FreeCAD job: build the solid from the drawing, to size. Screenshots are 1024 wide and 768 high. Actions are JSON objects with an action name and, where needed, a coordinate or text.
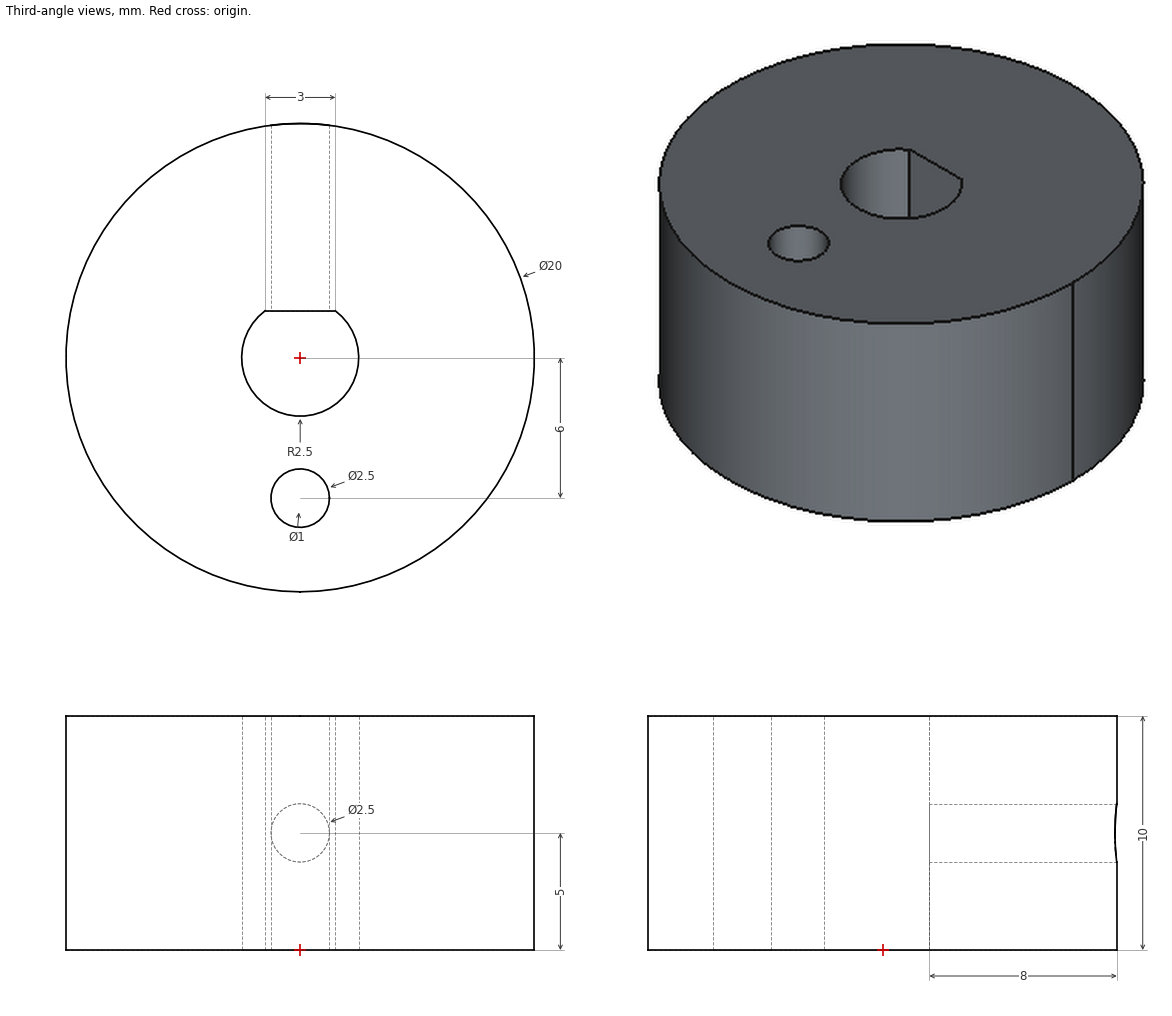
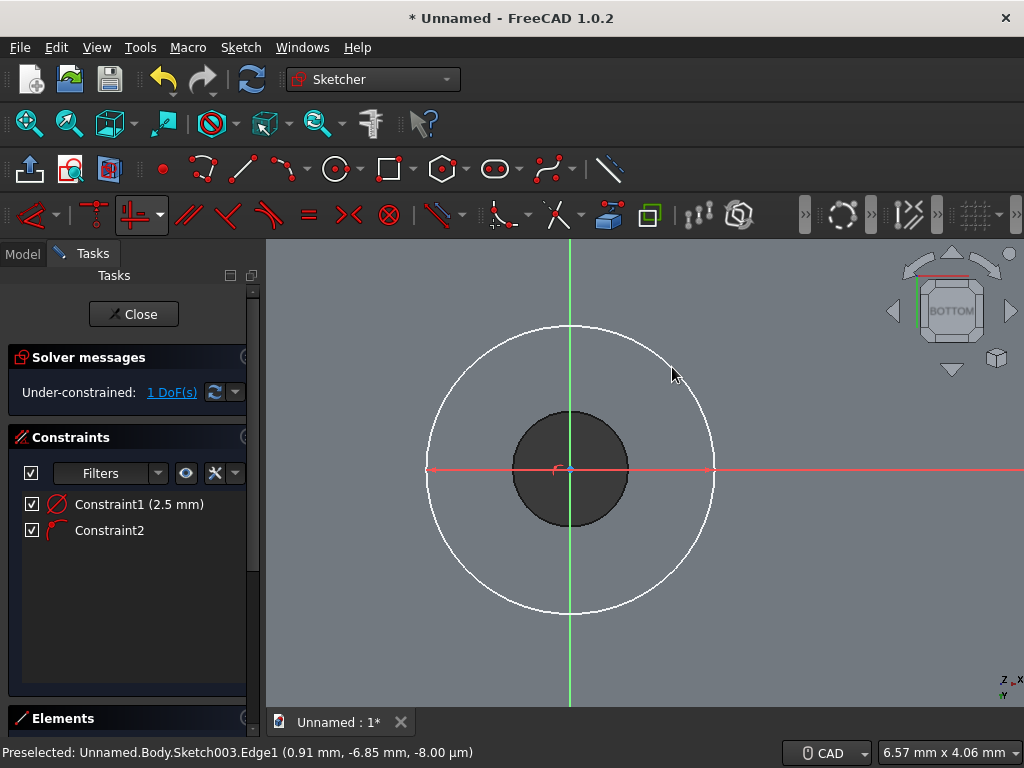
{"action": "left_click", "coordinate": [32, 216]}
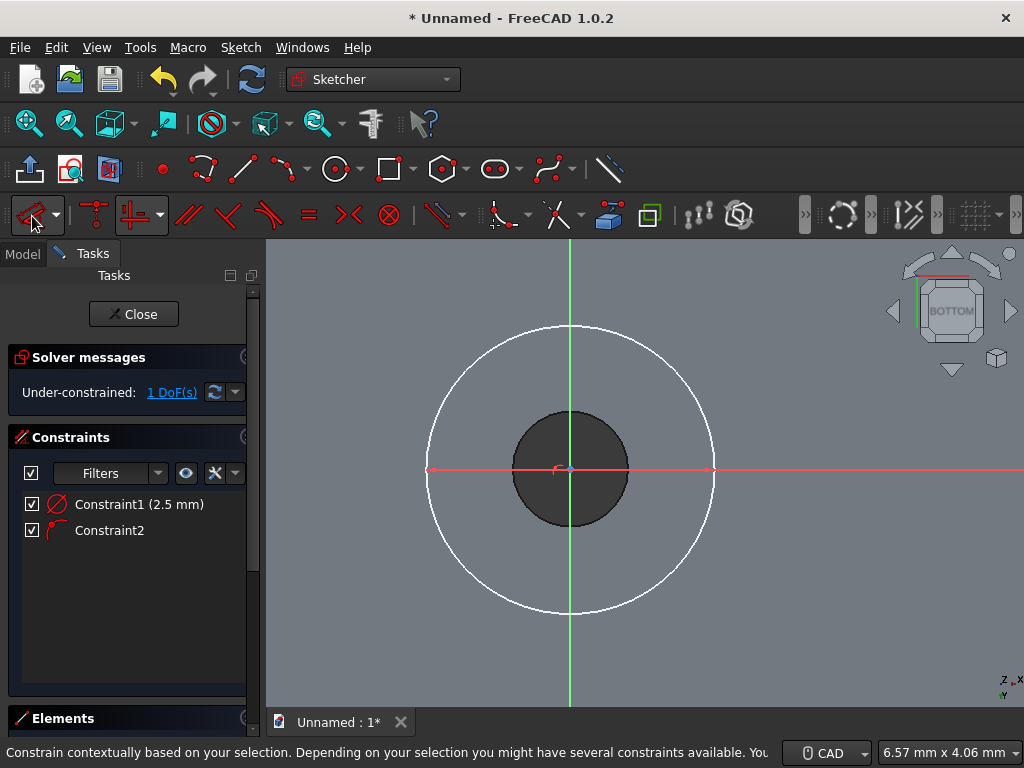
{"action": "left_click", "coordinate": [570, 470]}
{"action": "left_click", "coordinate": [604, 574]}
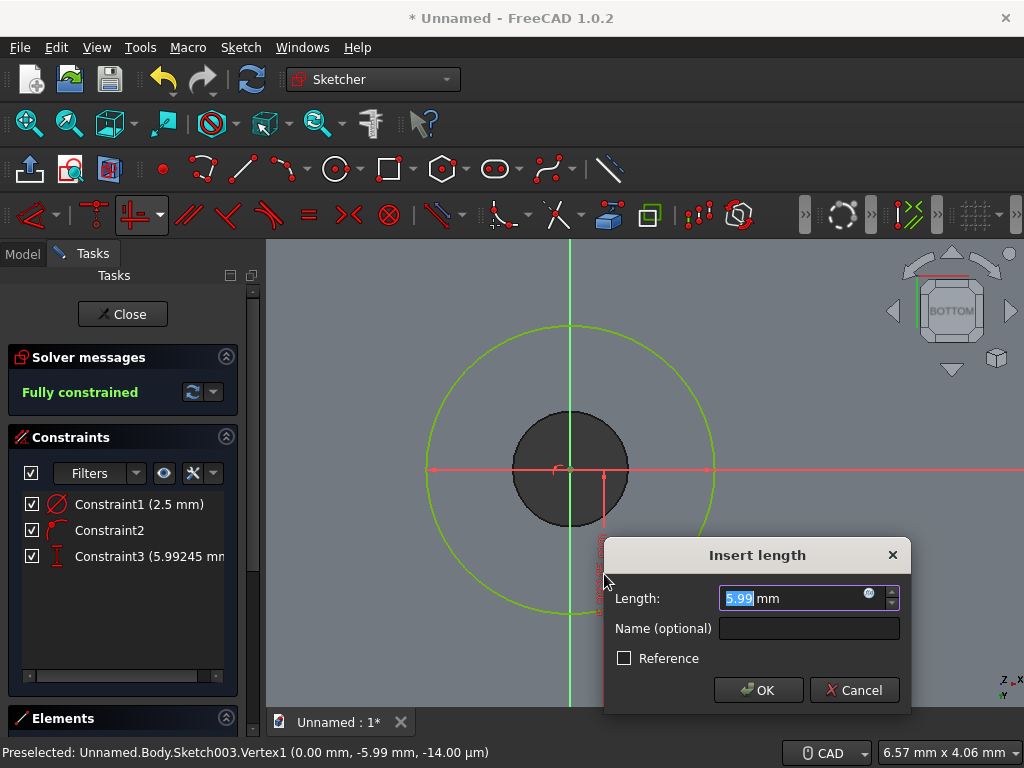
{"action": "type", "text": "6"}
{"action": "key", "text": "Return"}
{"action": "key", "text": "Escape"}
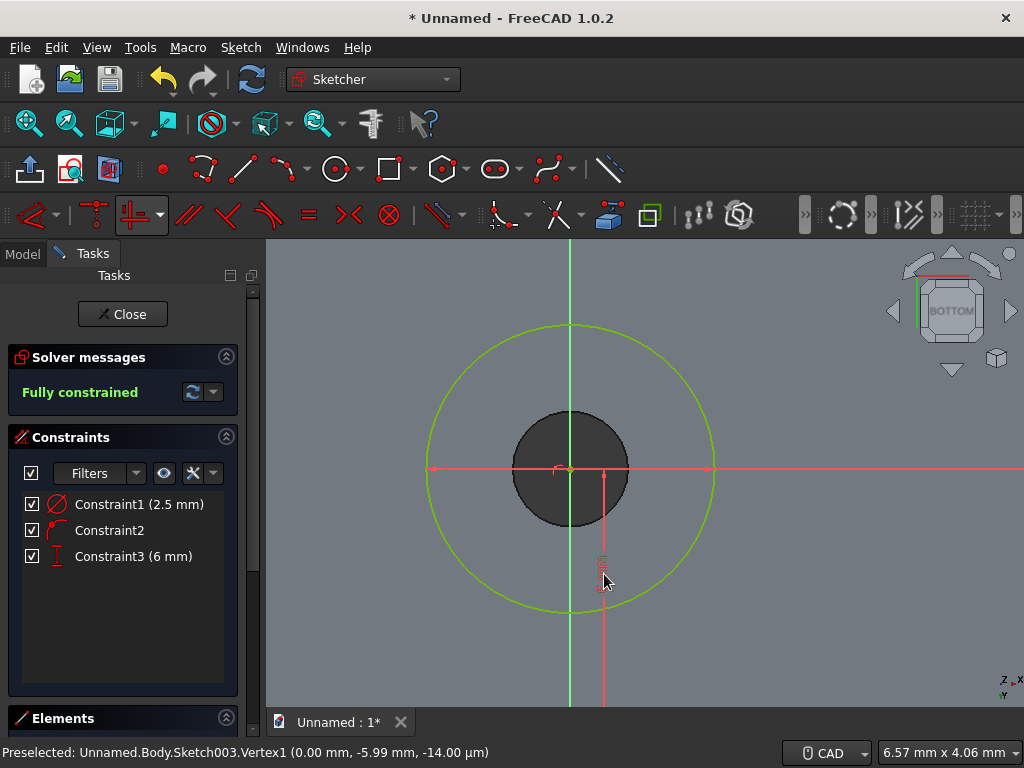
{"action": "left_click", "coordinate": [123, 314]}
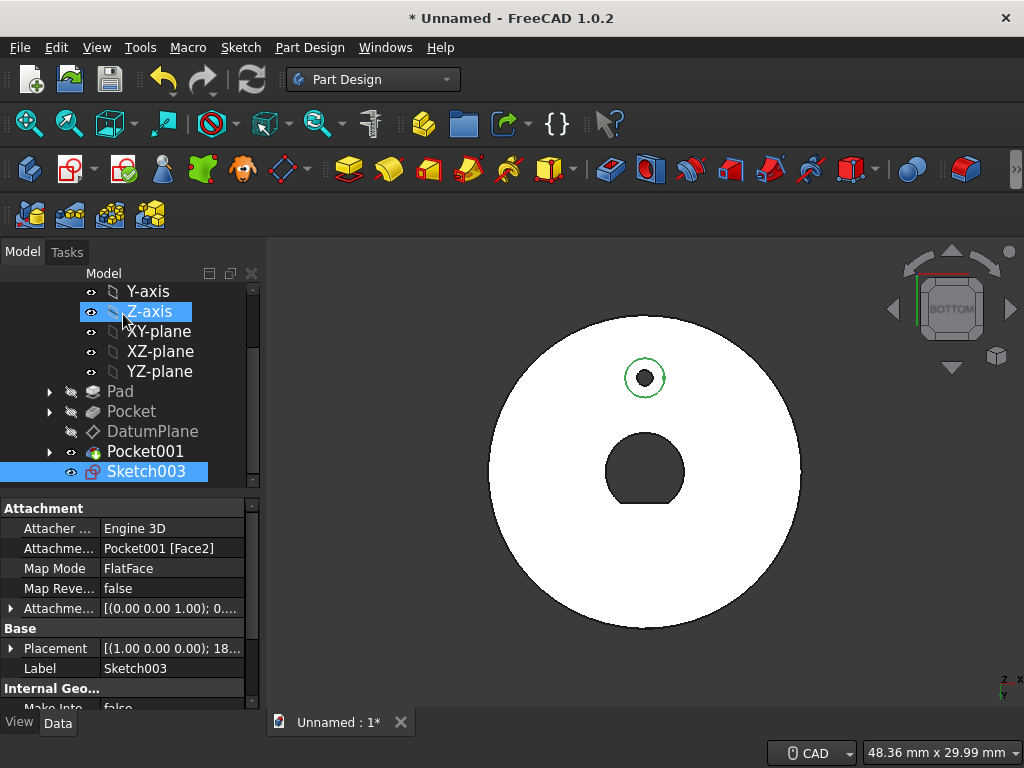
{"action": "left_click", "coordinate": [612, 170]}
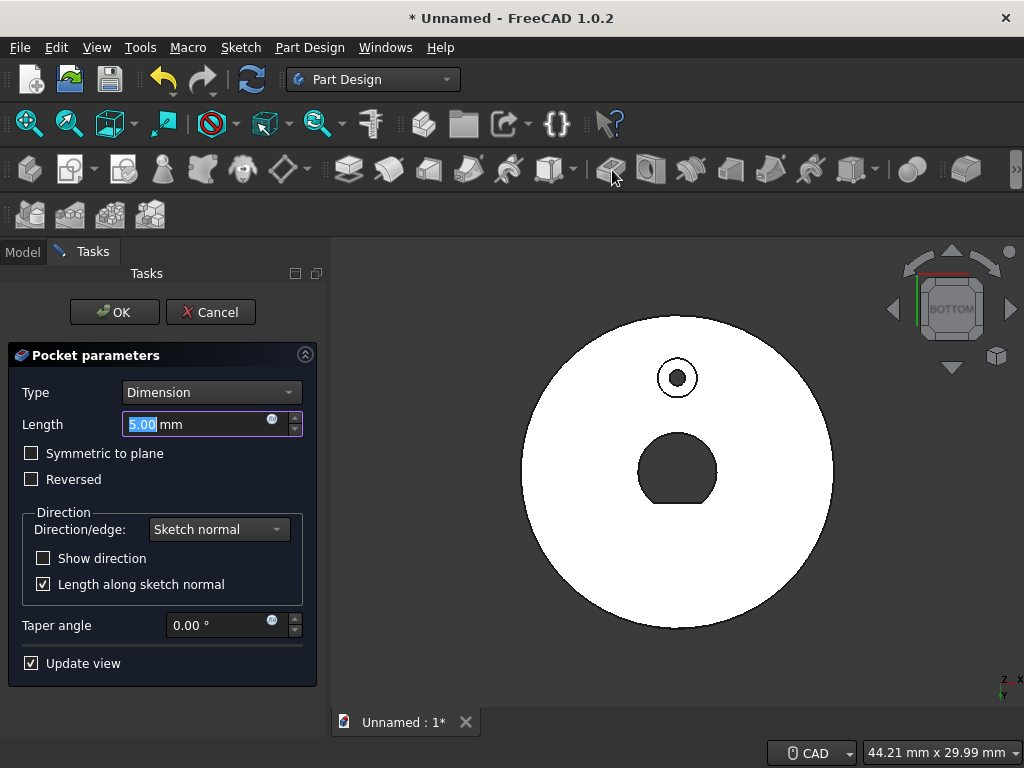
{"action": "left_click", "coordinate": [212, 392]}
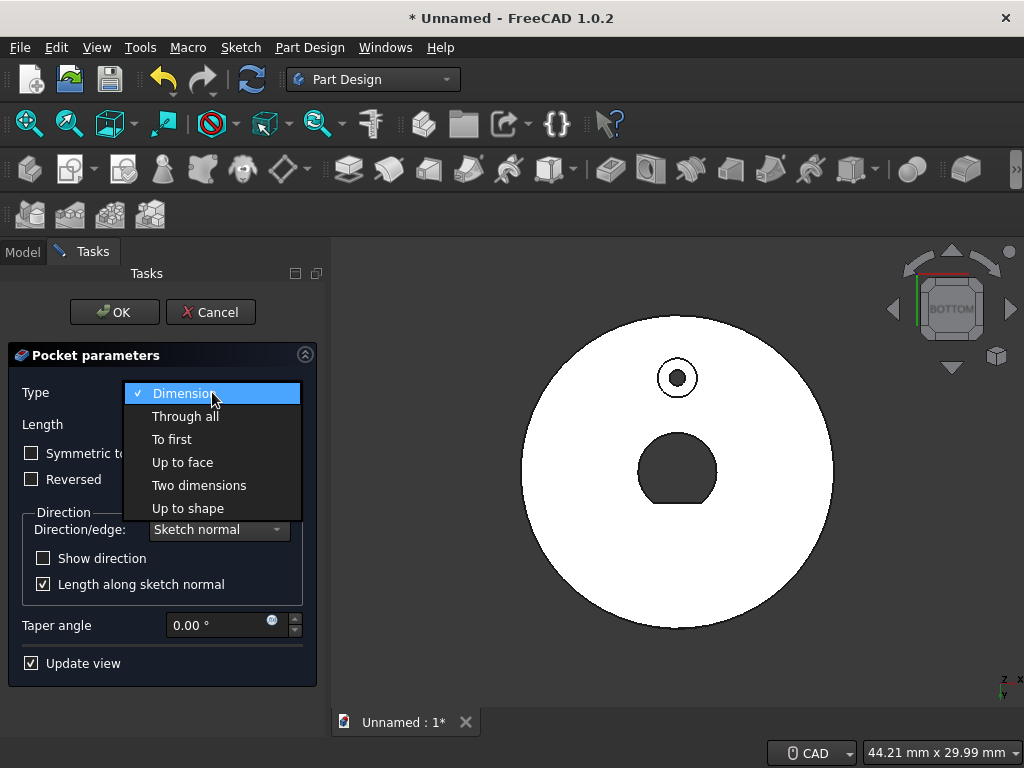
{"action": "left_click", "coordinate": [212, 416]}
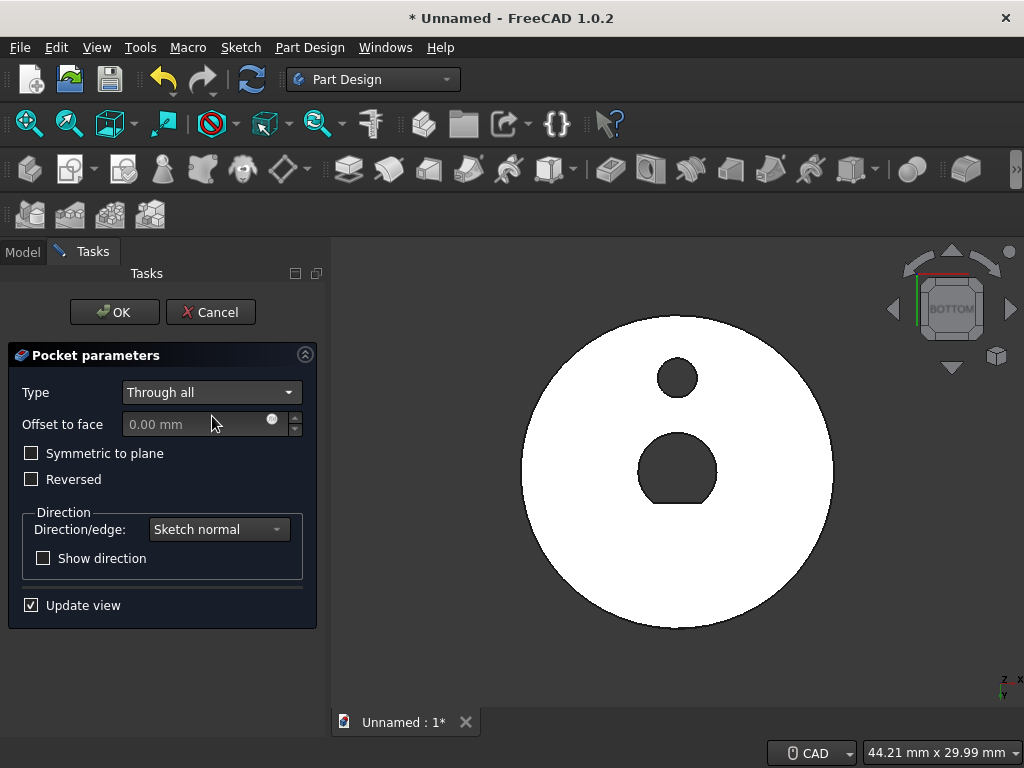
{"action": "left_click", "coordinate": [115, 312]}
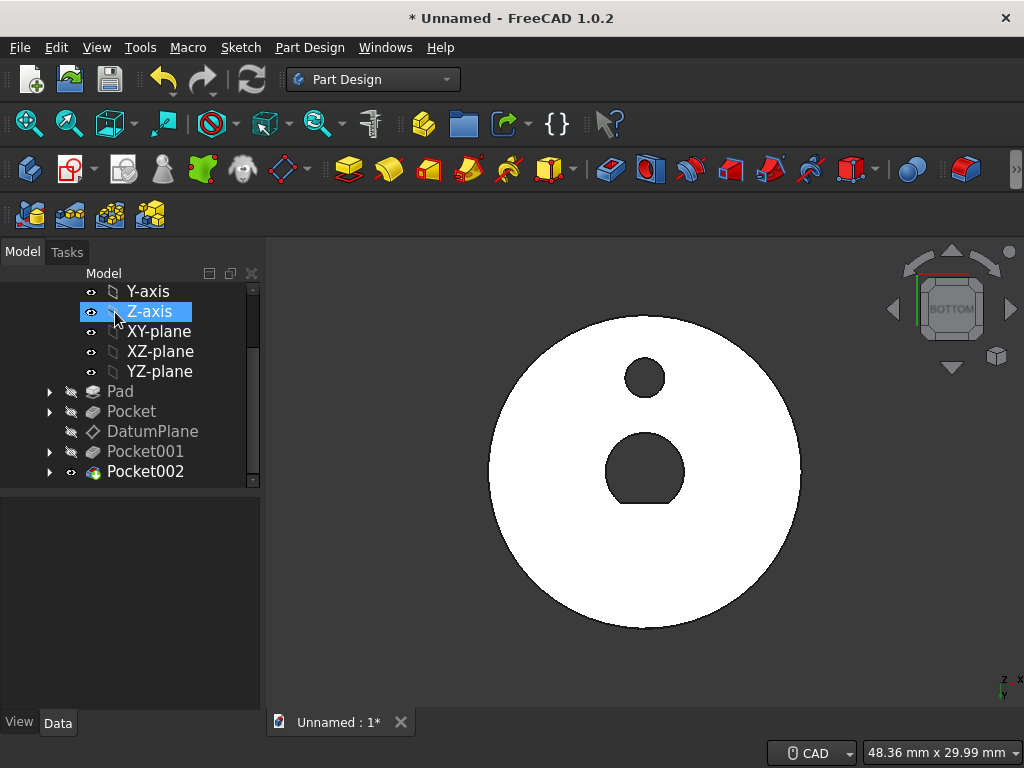
{"action": "key", "text": "0"}